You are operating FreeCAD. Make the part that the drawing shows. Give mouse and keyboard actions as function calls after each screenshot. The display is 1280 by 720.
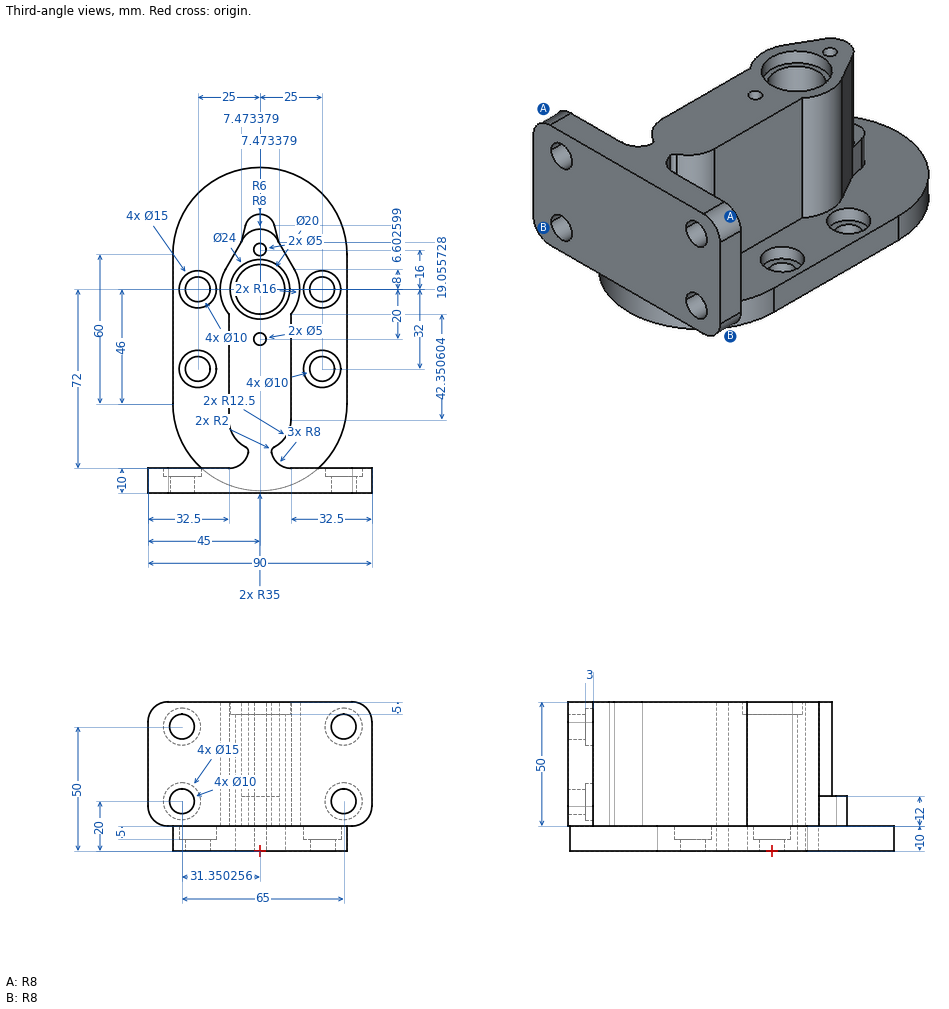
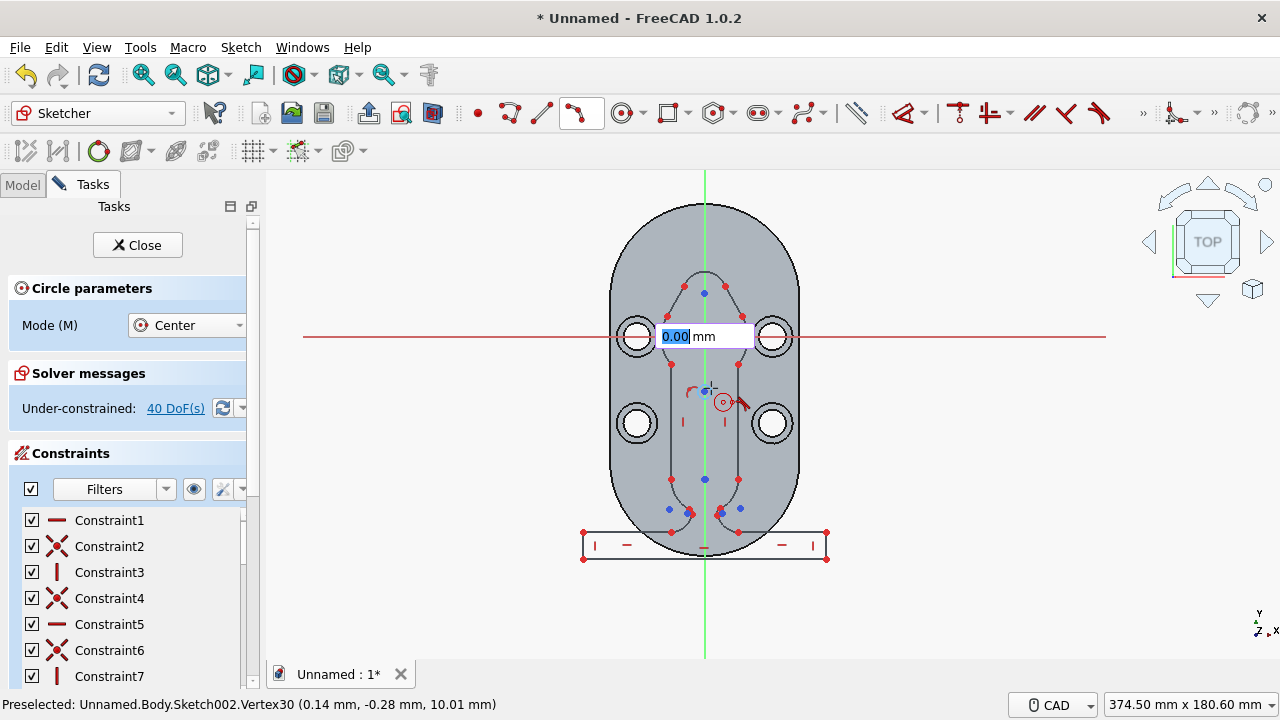
click(724, 318)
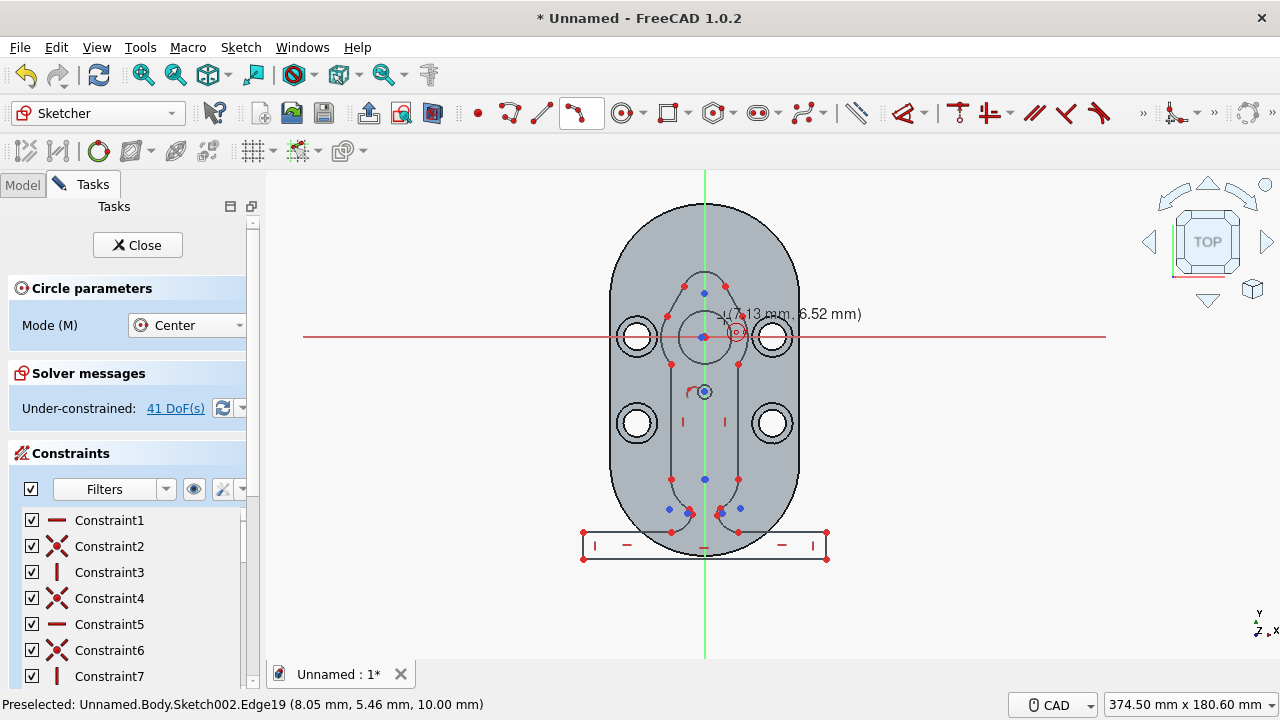
scroll(705, 293, up, 17)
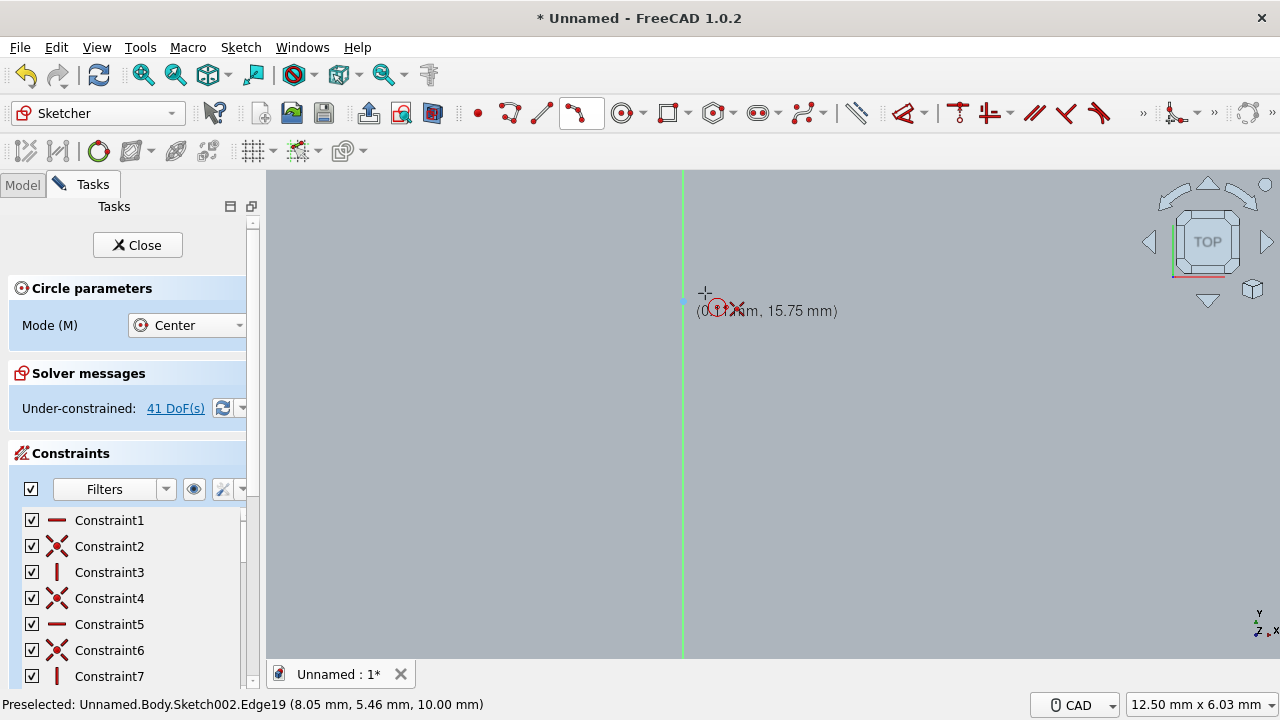
click(683, 295)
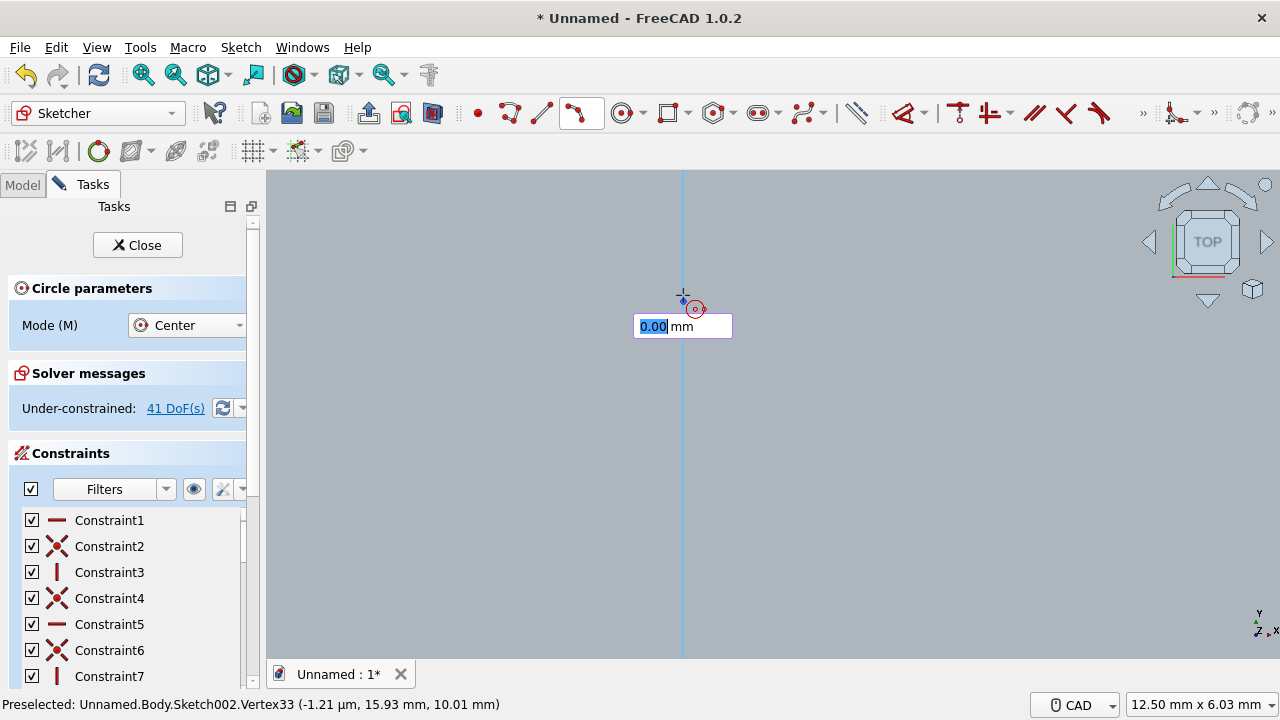
scroll(705, 265, down, 16)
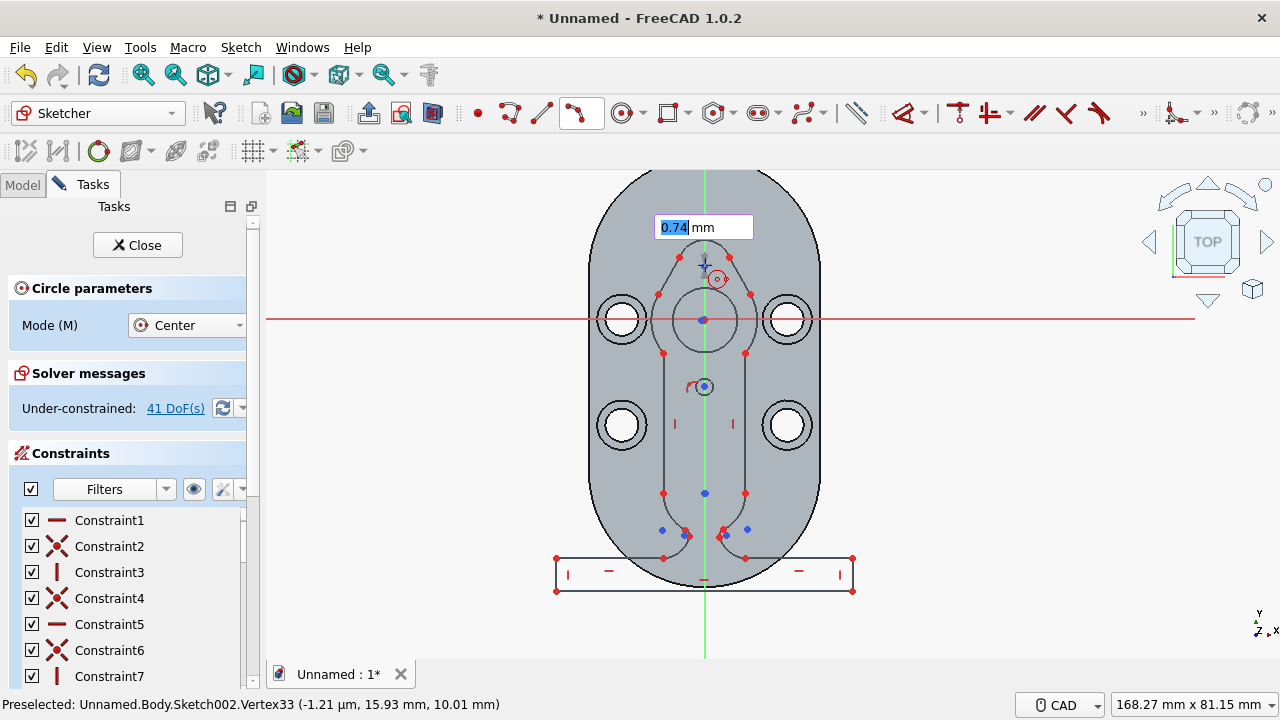
scroll(710, 261, up, 5)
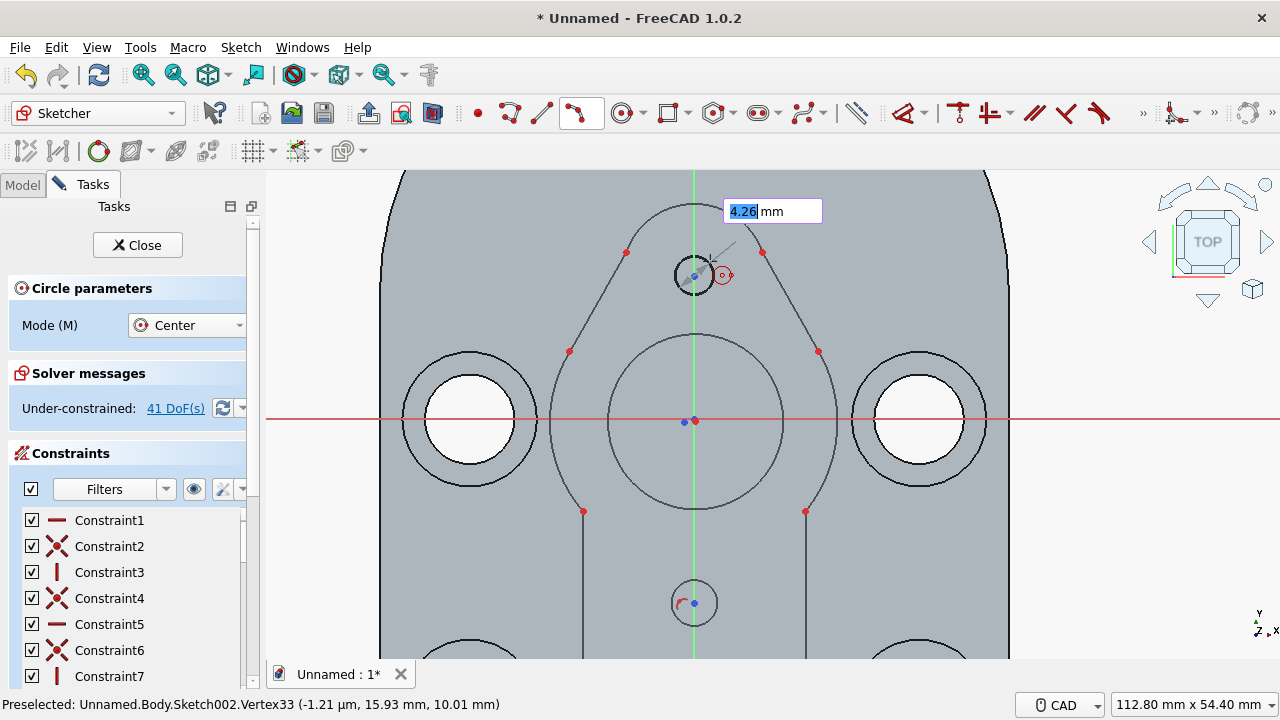
click(710, 260)
key(Escape)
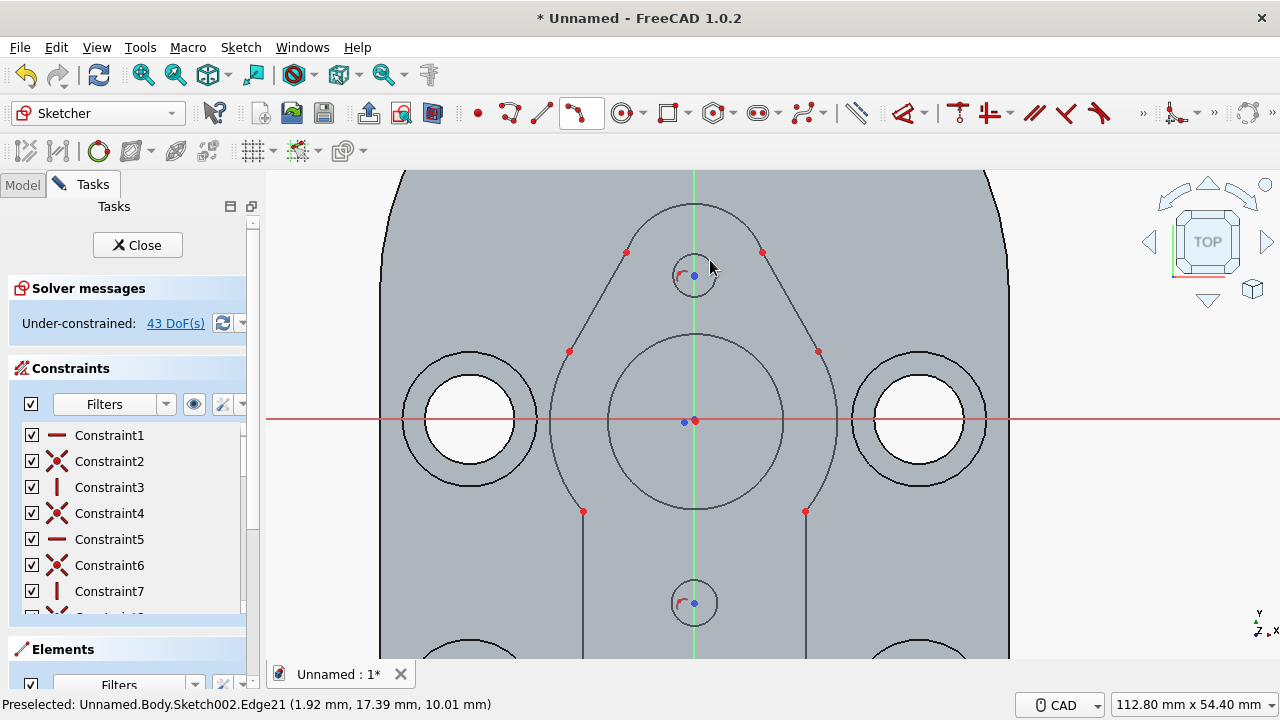
scroll(709, 300, down, 6)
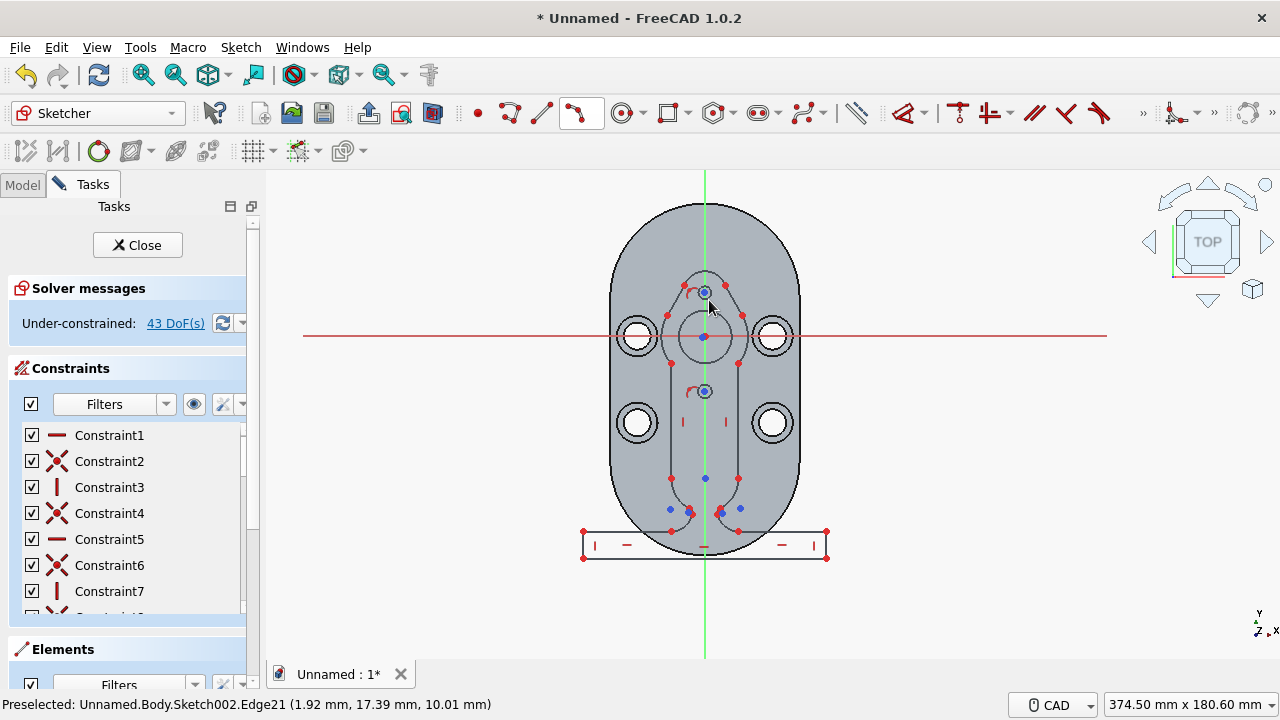
click(645, 532)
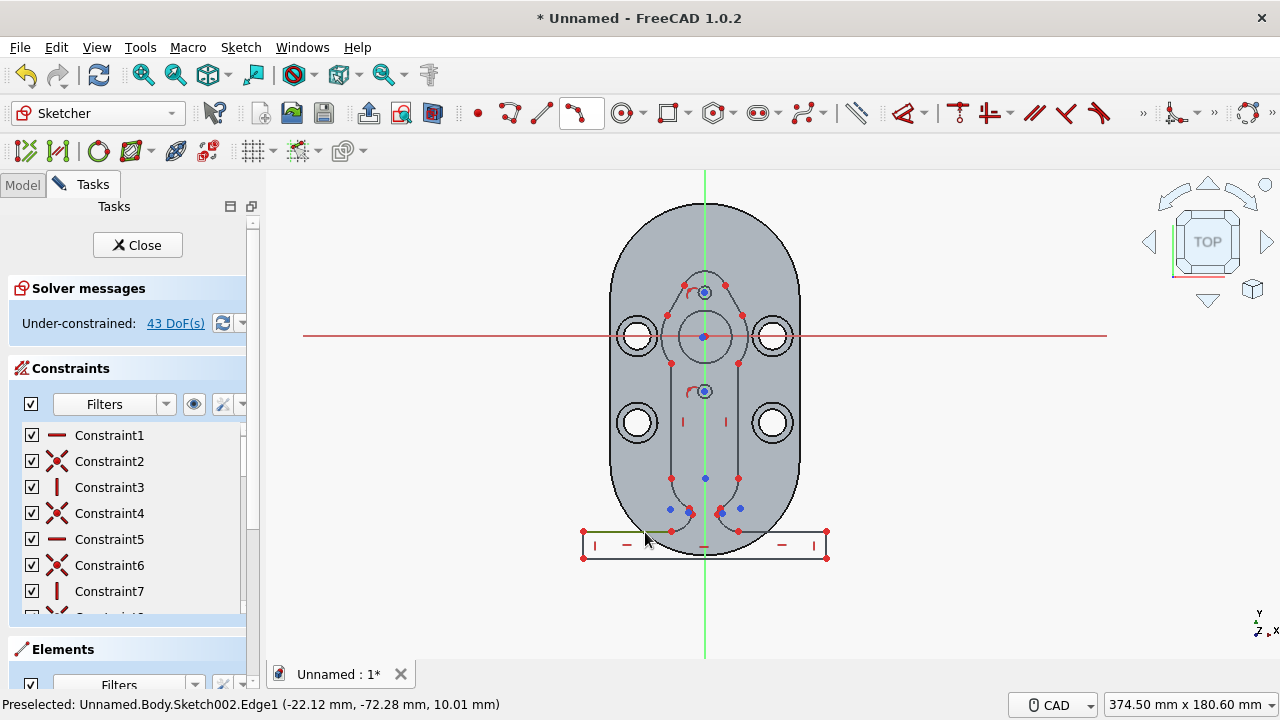
click(685, 526)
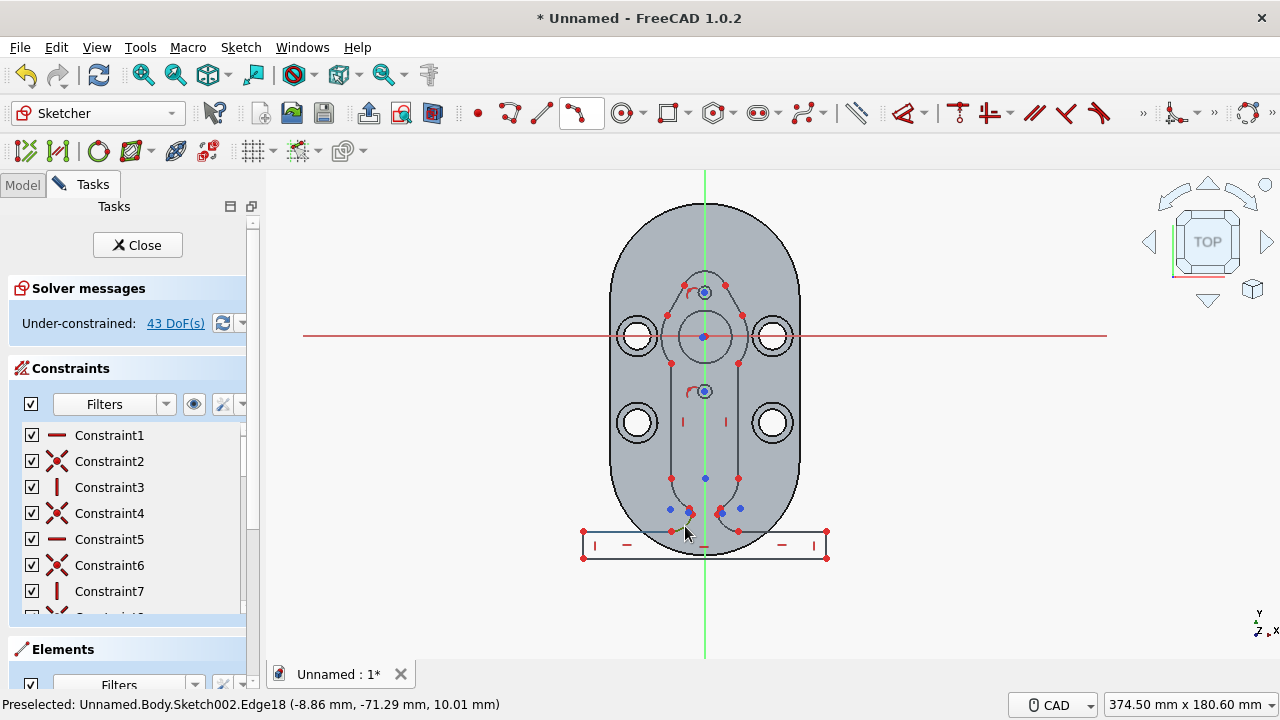
click(1100, 114)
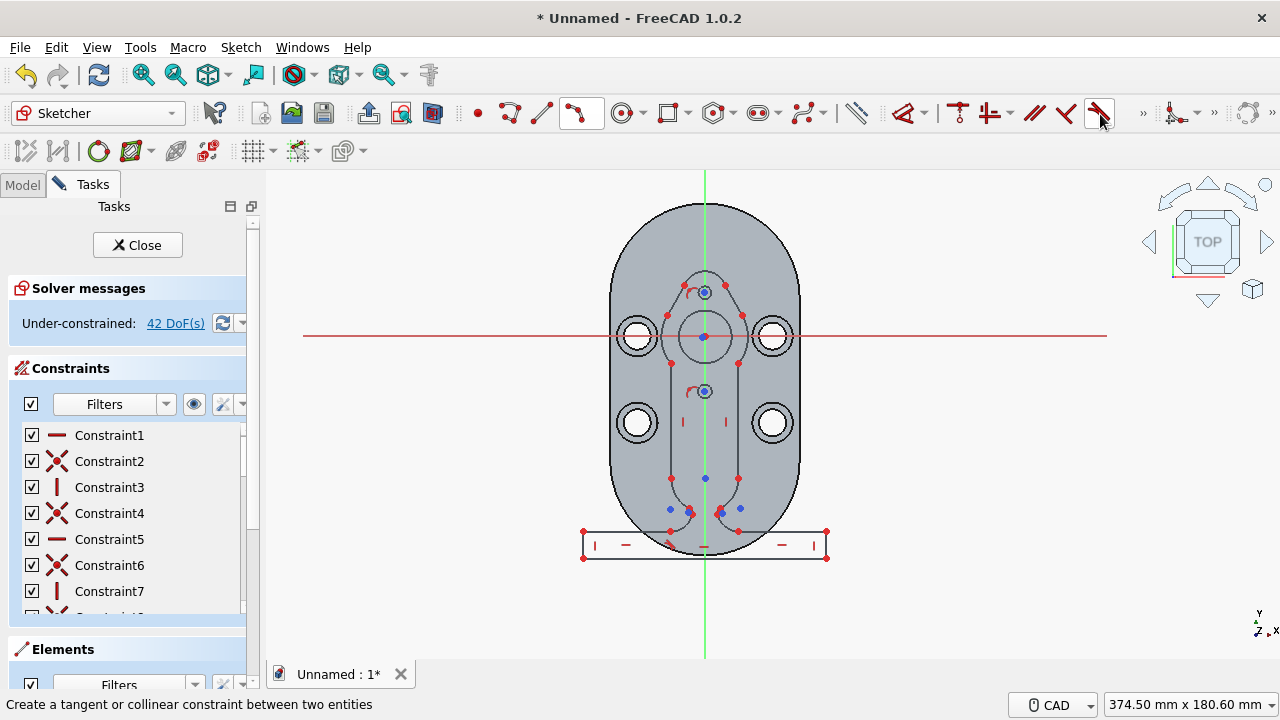
click(800, 532)